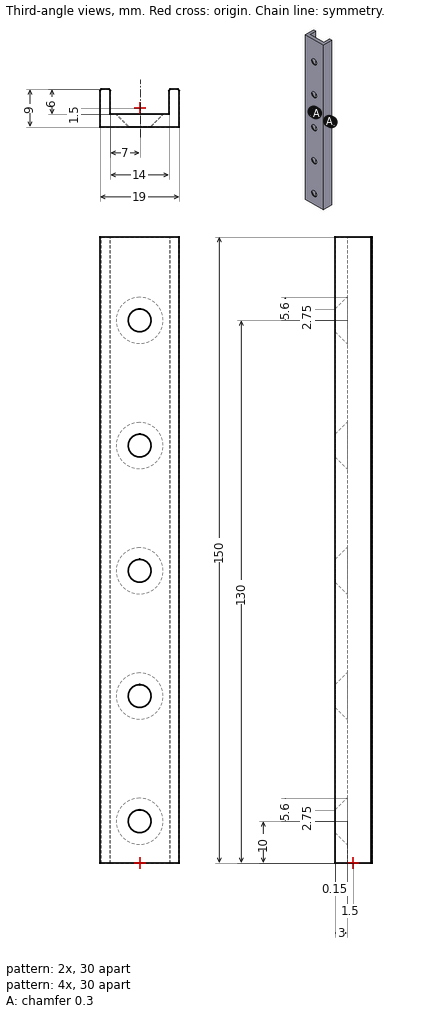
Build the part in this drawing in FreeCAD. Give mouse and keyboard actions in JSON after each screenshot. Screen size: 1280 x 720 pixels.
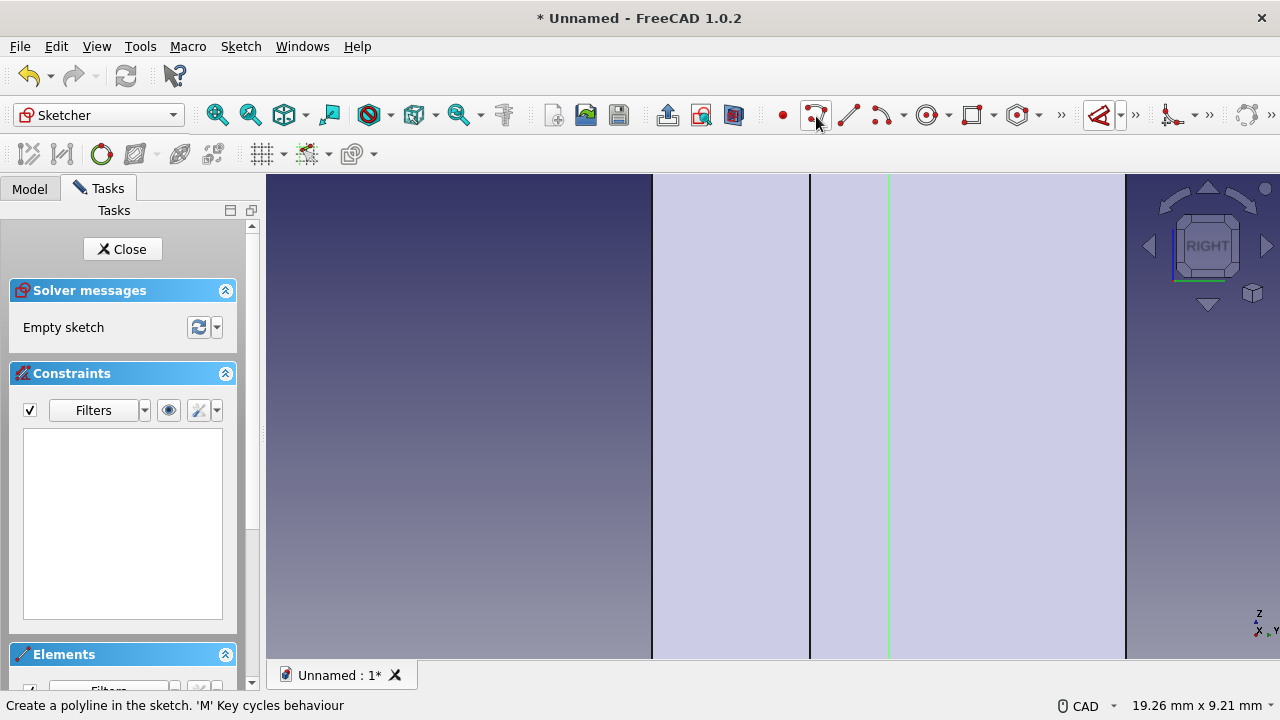
{"action": "left_click", "coordinate": [810, 543]}
{"action": "left_click", "coordinate": [810, 248]}
{"action": "left_click", "coordinate": [660, 398]}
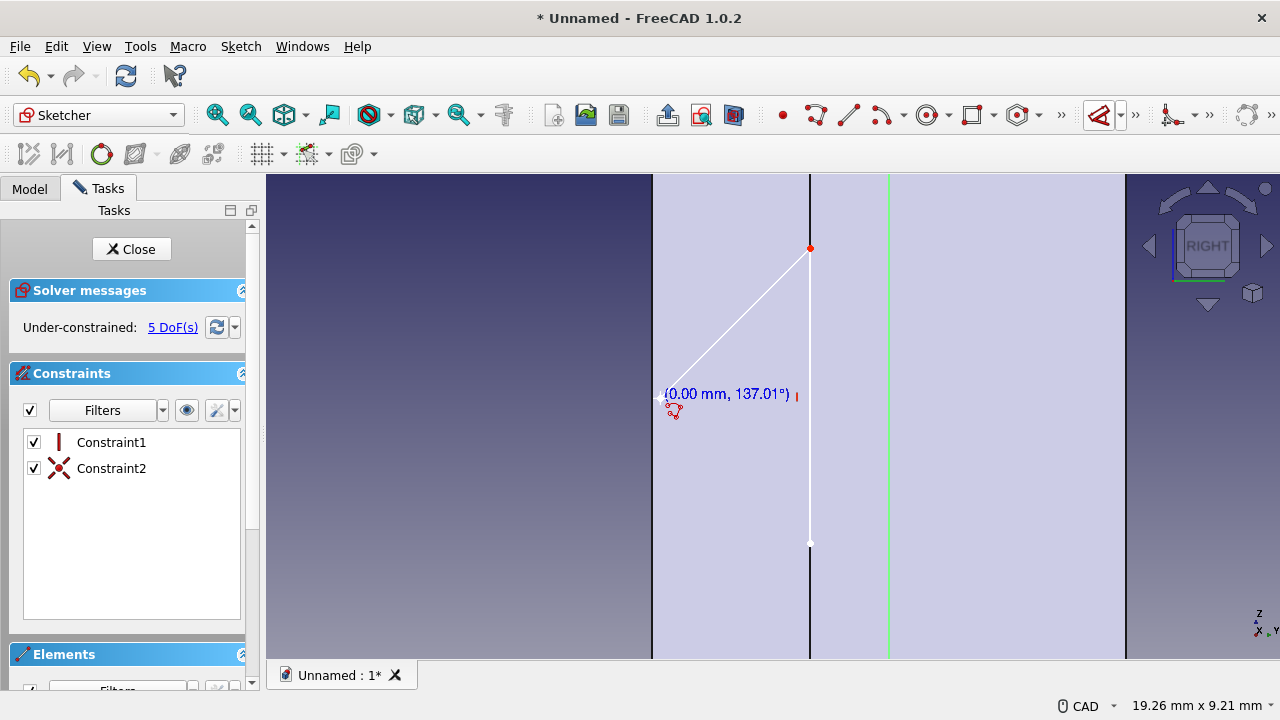
{"action": "scroll", "coordinate": [652, 398], "scroll_direction": "up", "scroll_amount": 4}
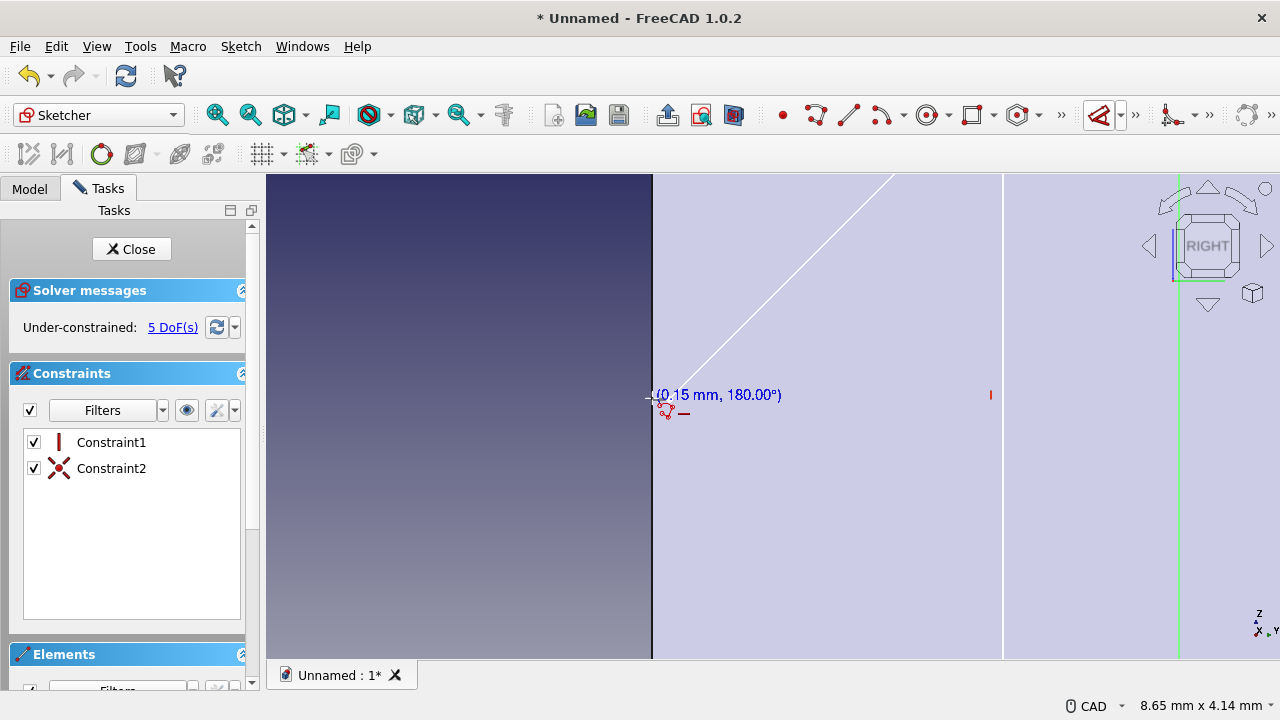
{"action": "left_click", "coordinate": [652, 397]}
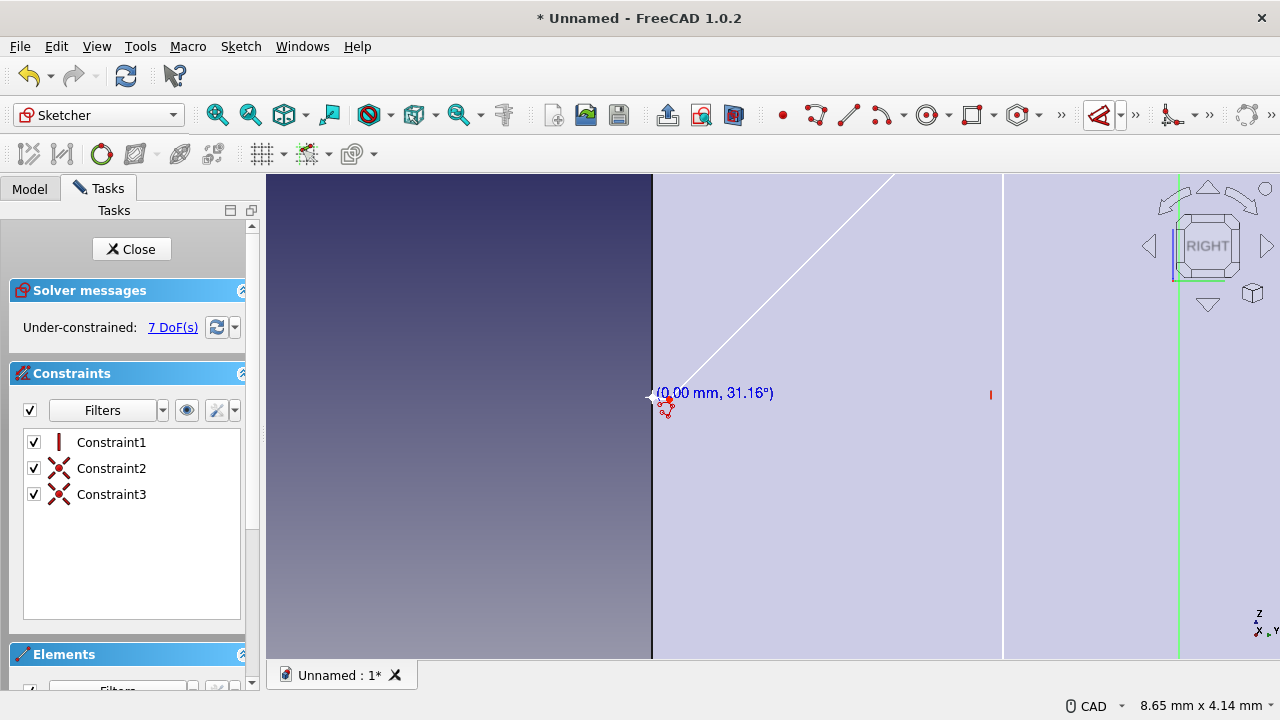
{"action": "scroll", "coordinate": [662, 437], "scroll_direction": "down", "scroll_amount": 4}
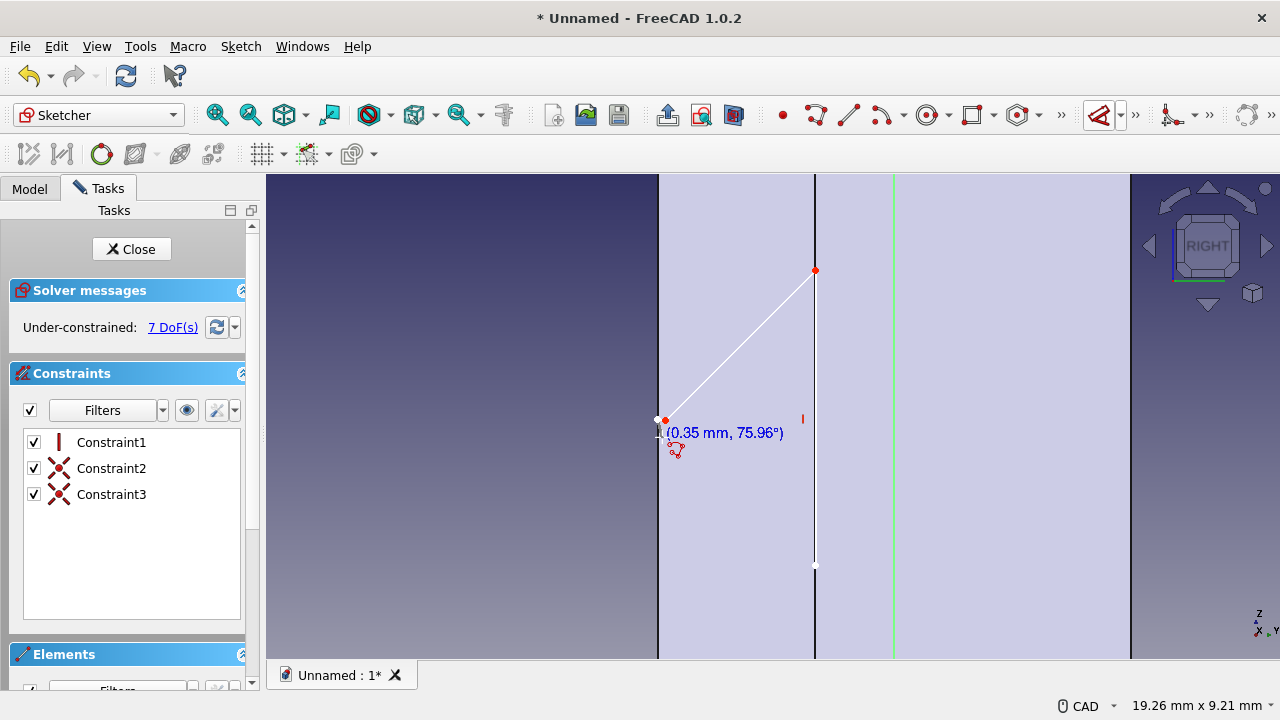
{"action": "left_click", "coordinate": [658, 564]}
{"action": "left_click", "coordinate": [816, 566]}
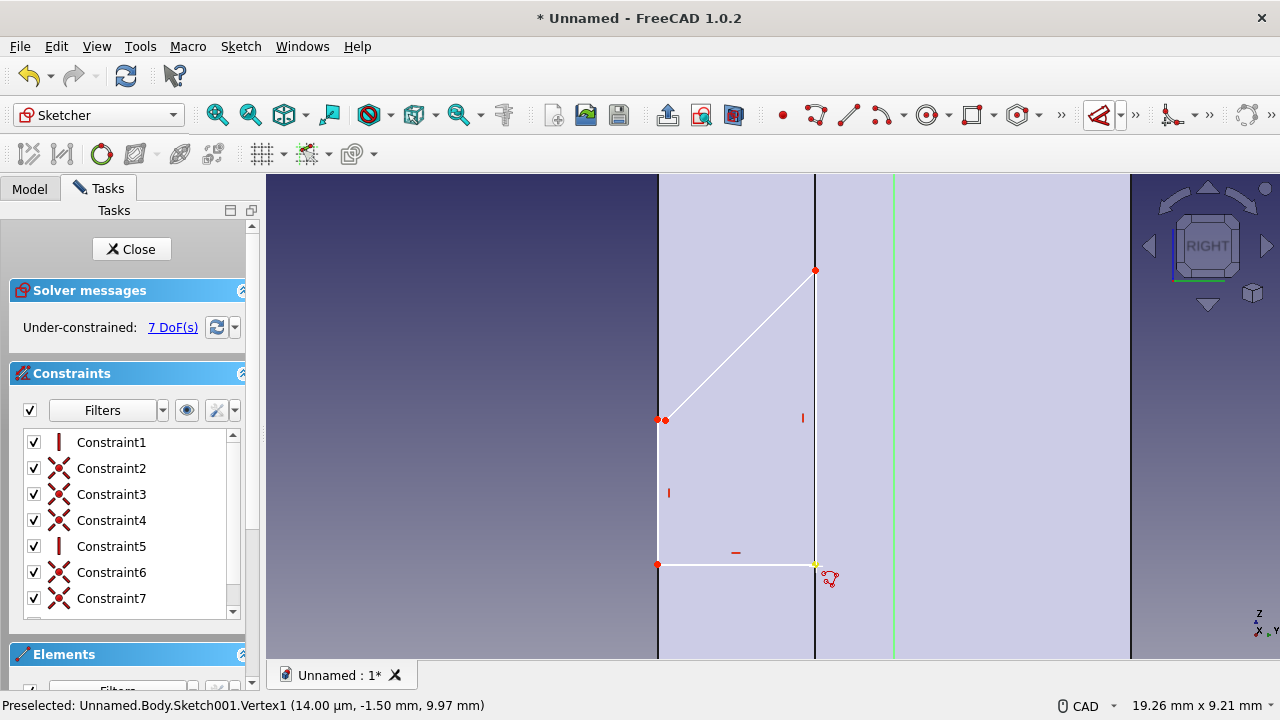
{"action": "left_click", "coordinate": [849, 116]}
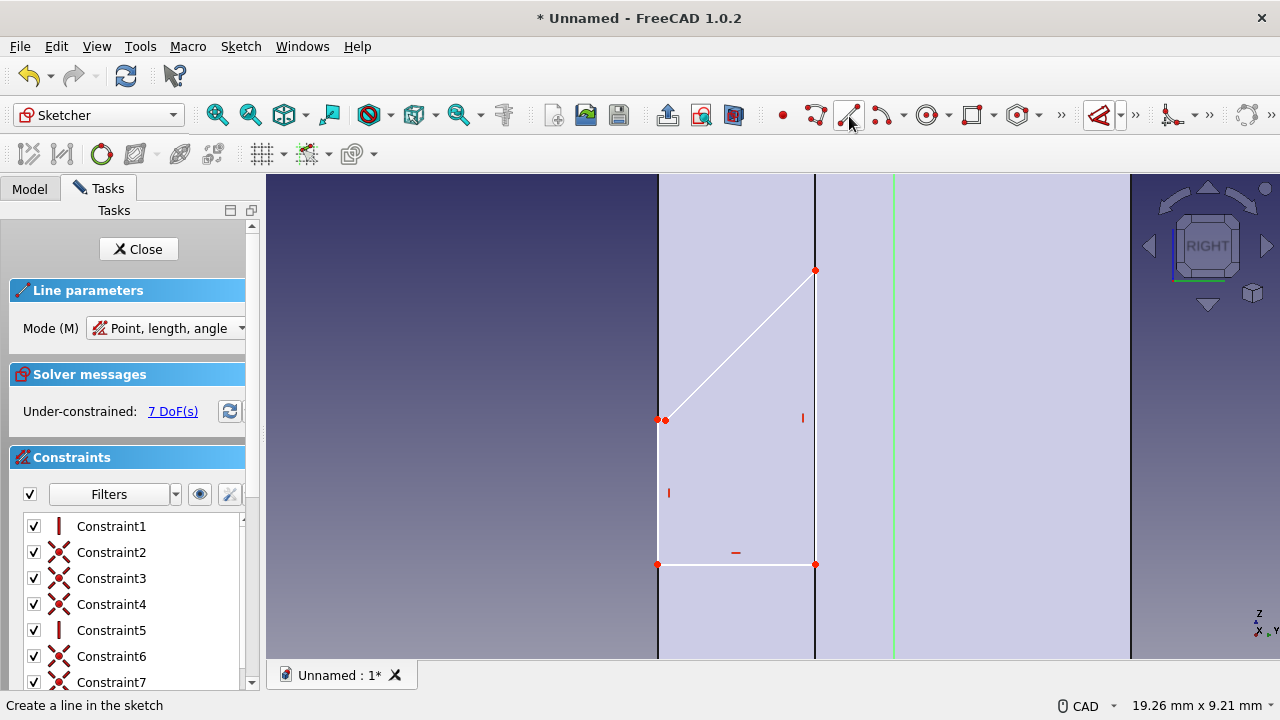
{"action": "left_click", "coordinate": [642, 564]}
{"action": "left_click", "coordinate": [594, 564]}
{"action": "key", "text": "Escape"}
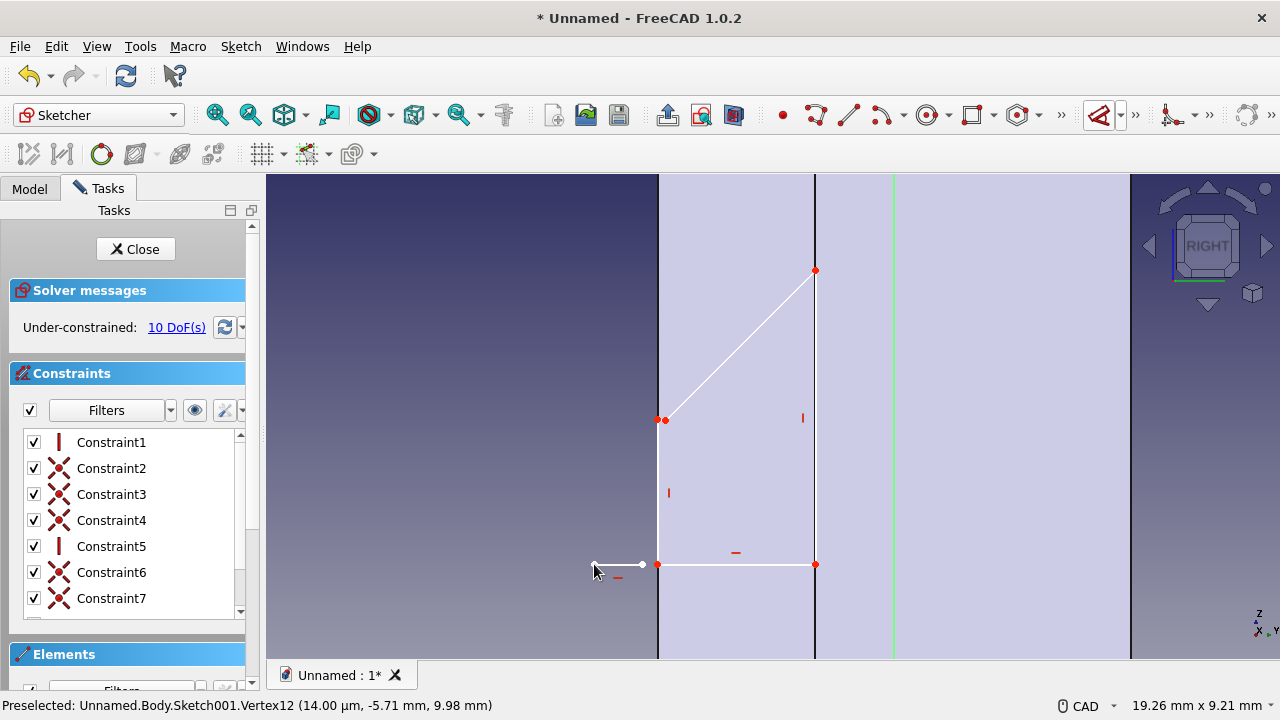
{"action": "left_click", "coordinate": [628, 565]}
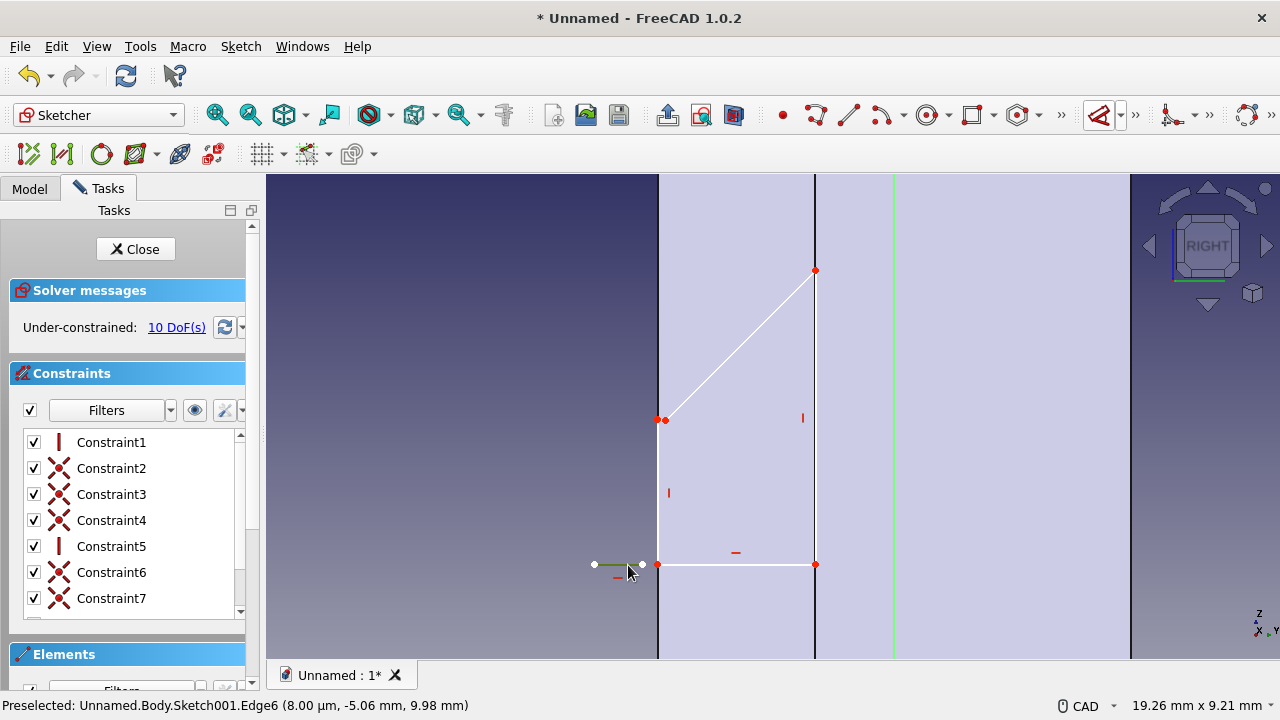
{"action": "key", "text": "g n"}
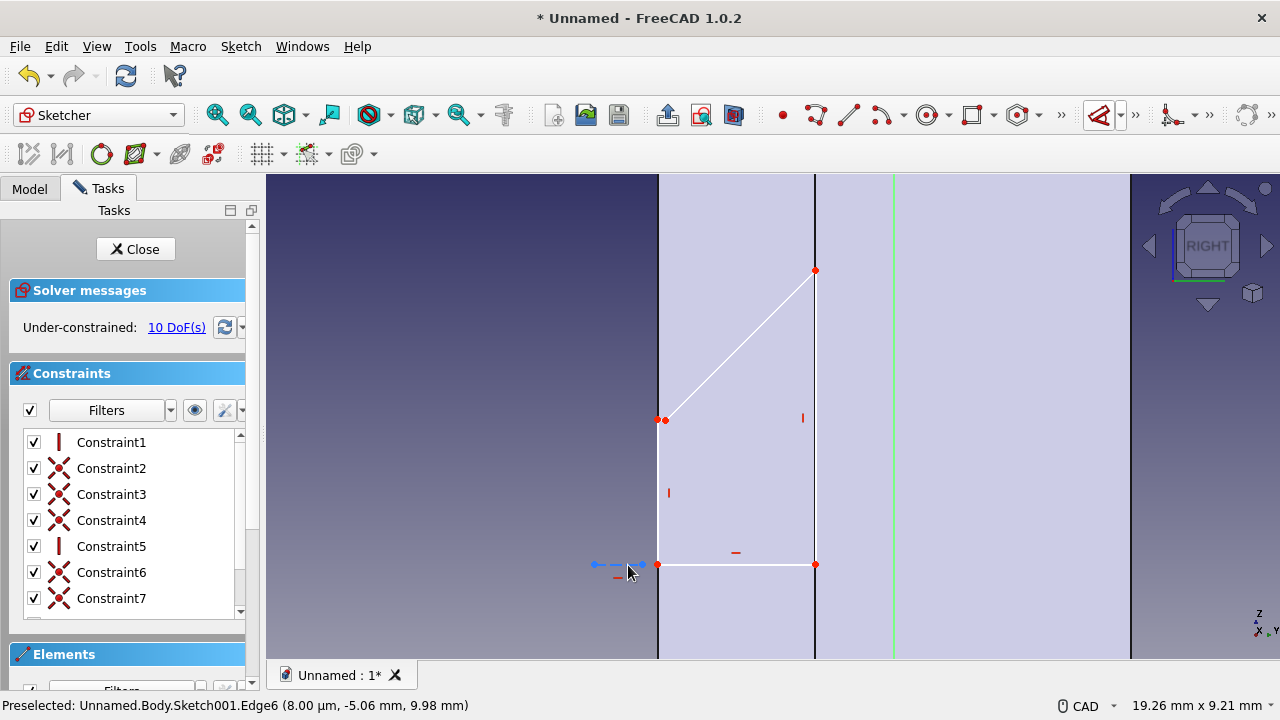
{"action": "scroll", "coordinate": [662, 420], "scroll_direction": "up", "scroll_amount": 7}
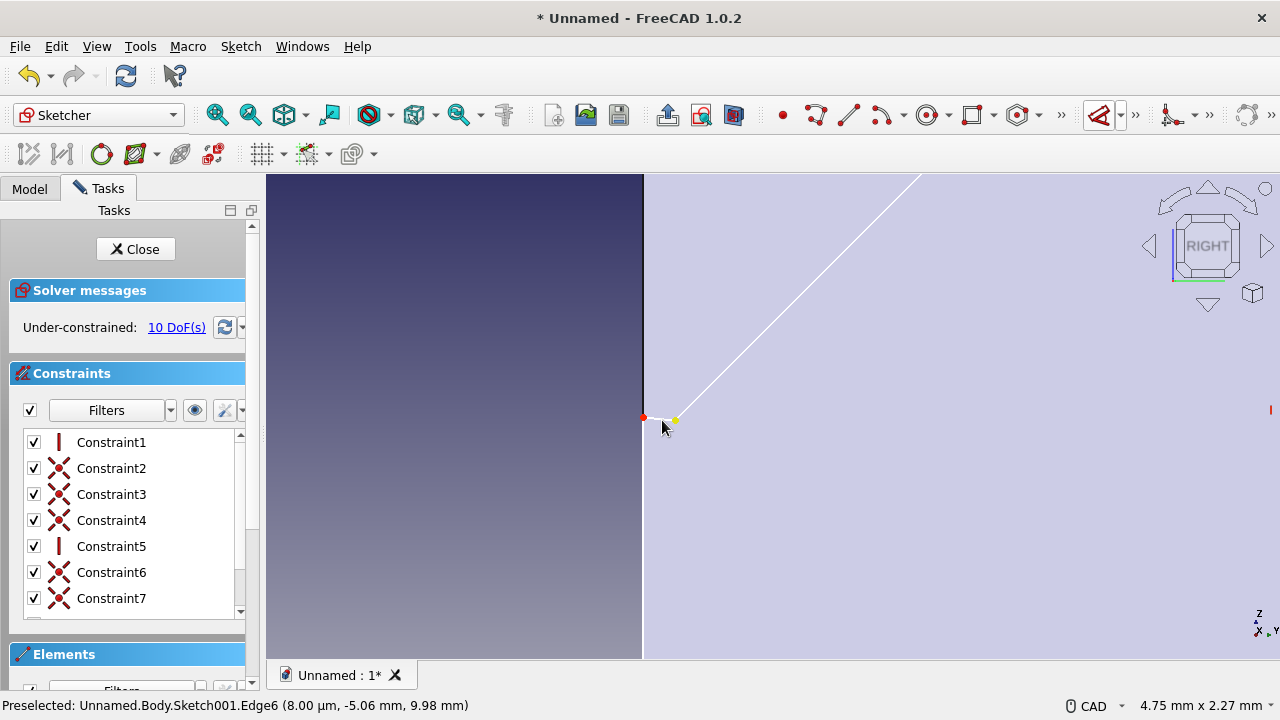
{"action": "left_click", "coordinate": [659, 419]}